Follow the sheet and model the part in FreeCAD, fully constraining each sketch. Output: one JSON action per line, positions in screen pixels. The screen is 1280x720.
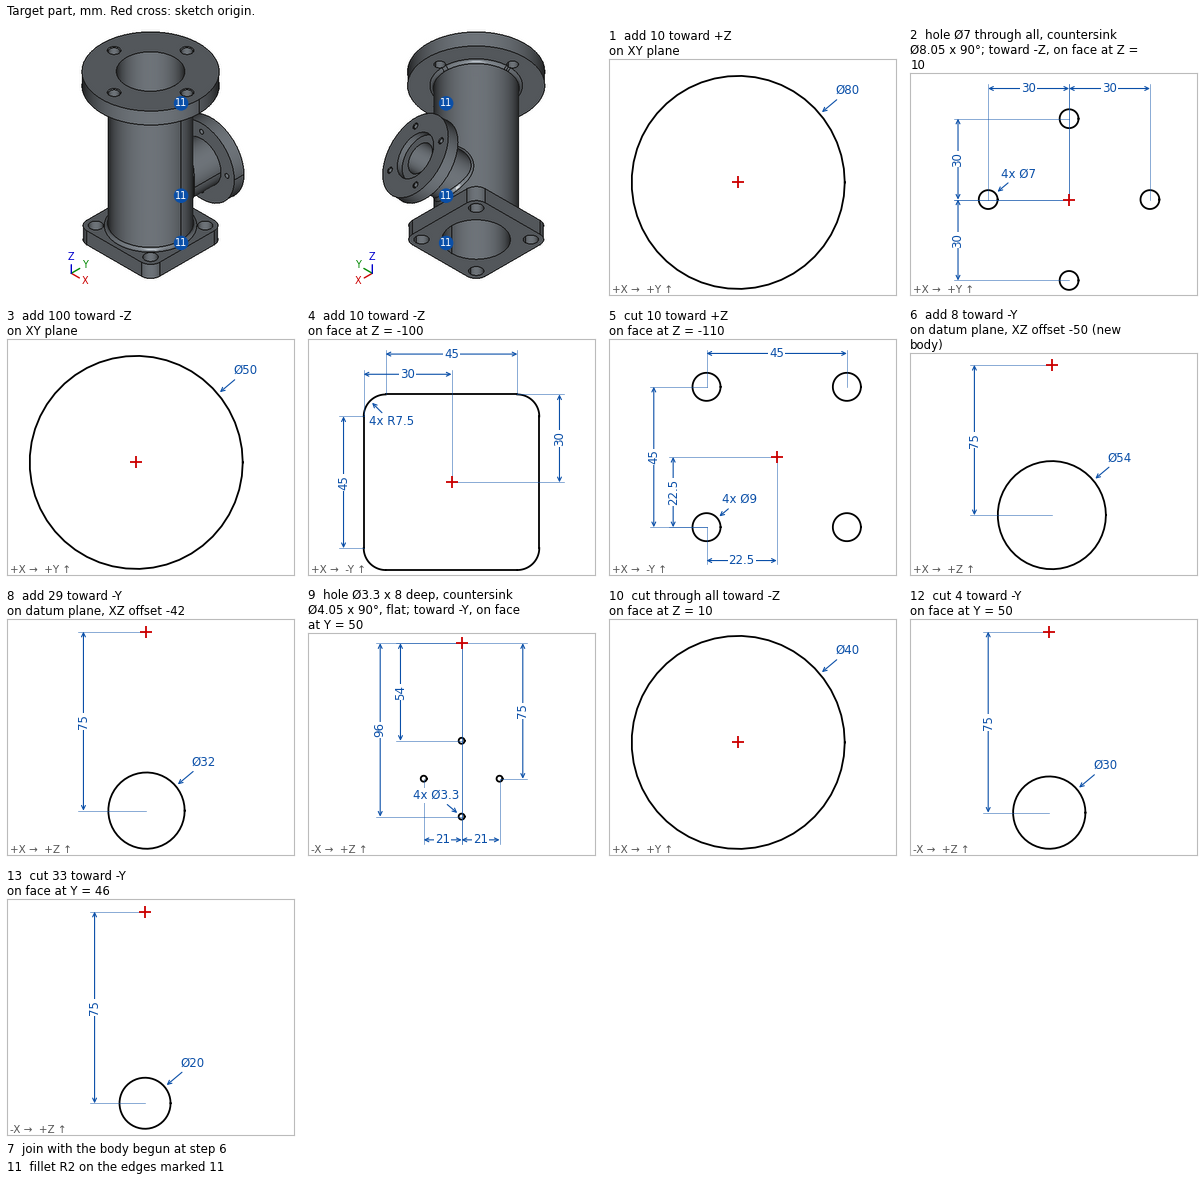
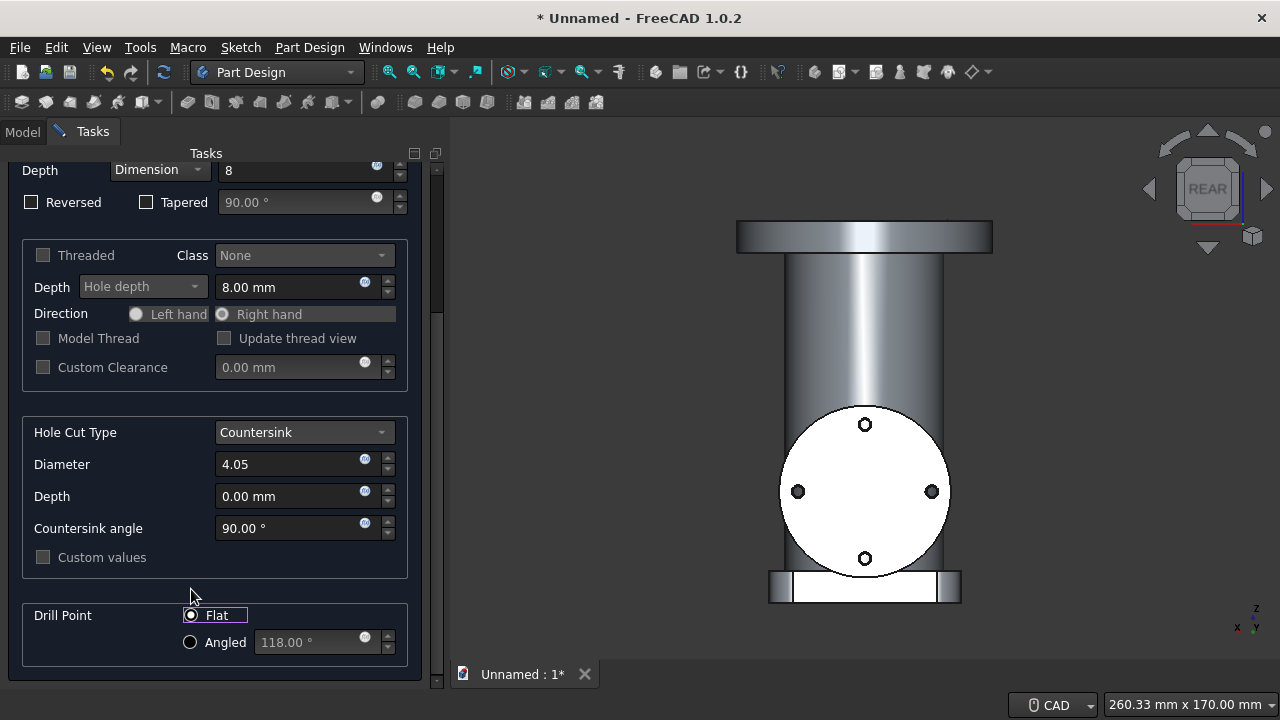
{"action": "scroll", "coordinate": [437, 426], "scroll_direction": "up", "scroll_amount": 5}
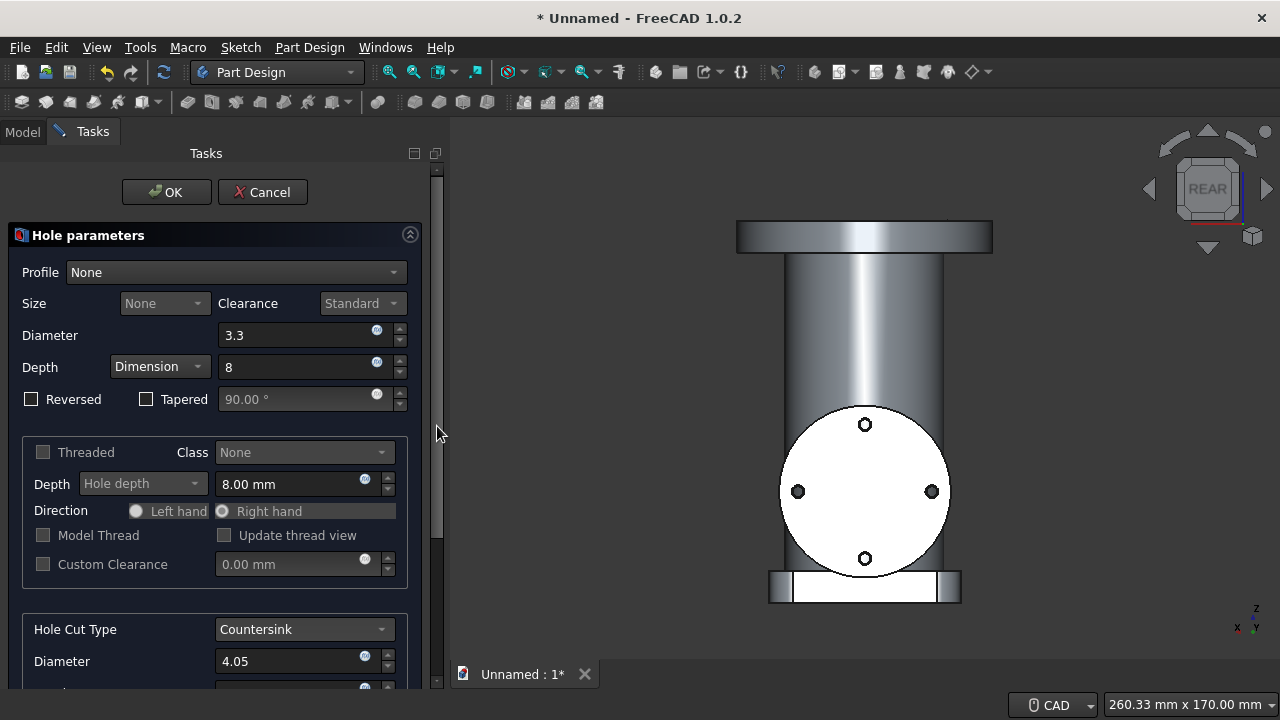
{"action": "left_click", "coordinate": [167, 192]}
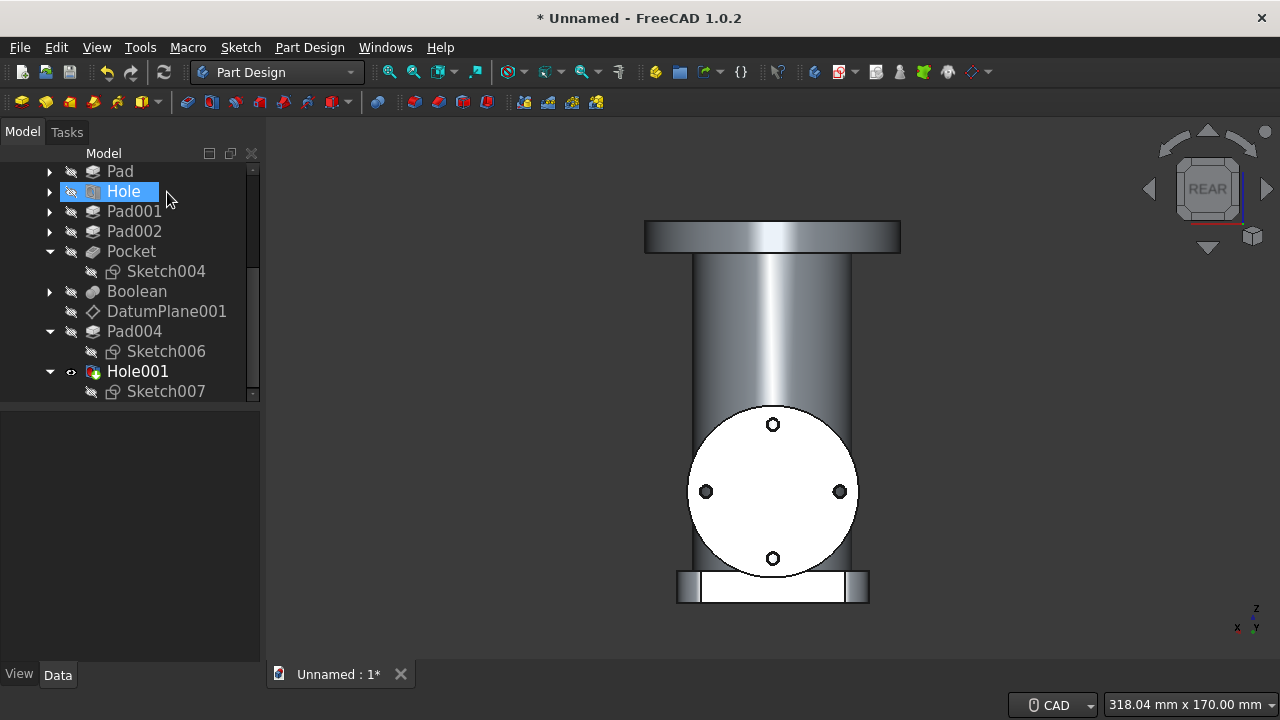
{"action": "key", "text": "0"}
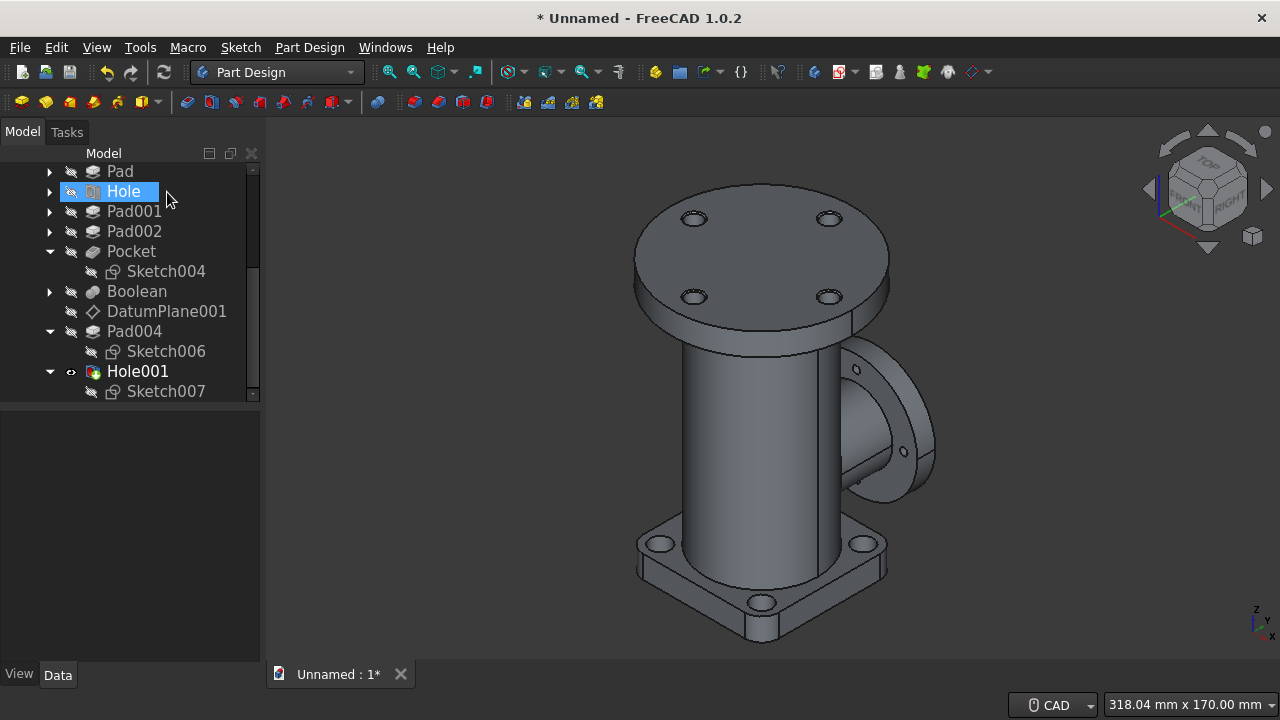
{"action": "left_click", "coordinate": [390, 72]}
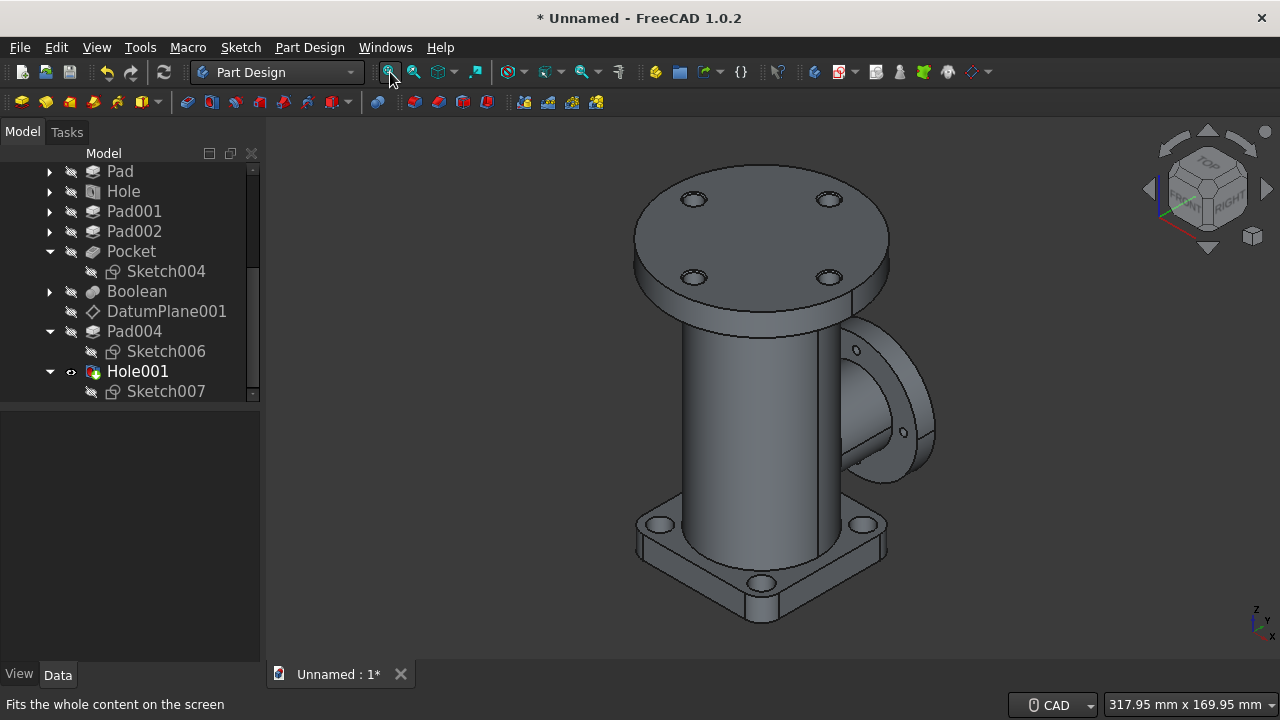
{"action": "left_click", "coordinate": [762, 237]}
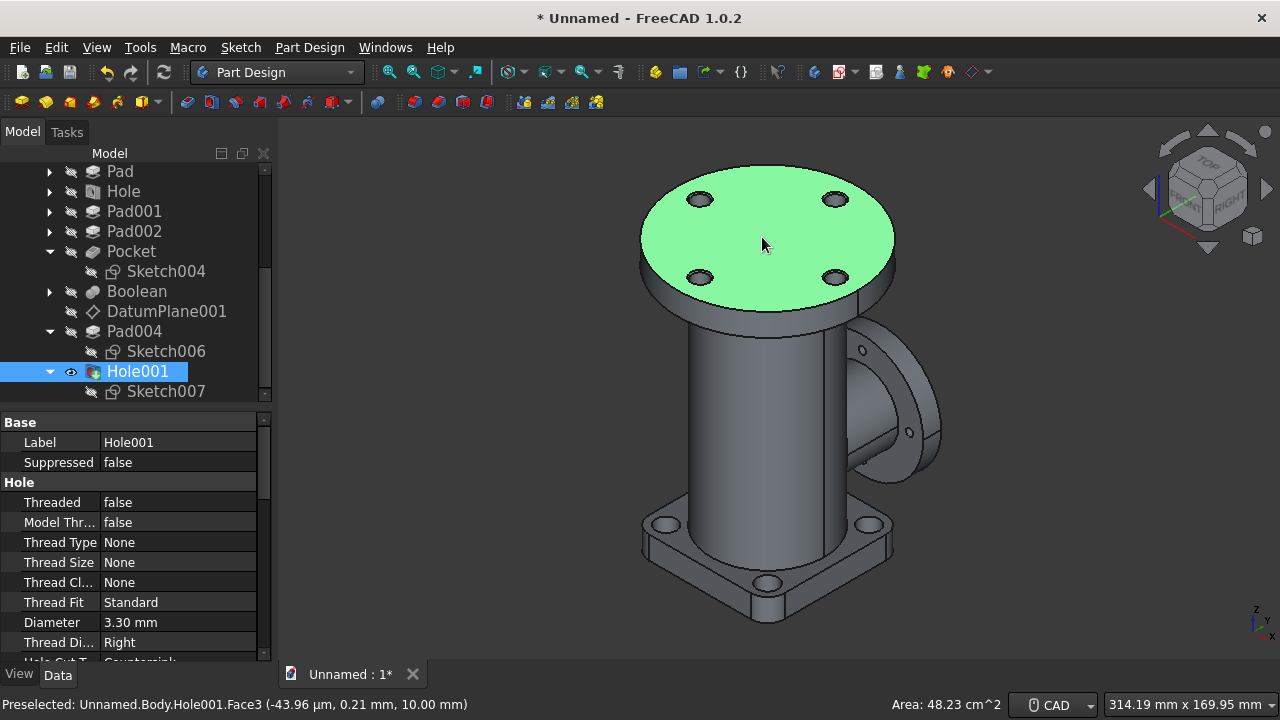
{"action": "left_click", "coordinate": [840, 72]}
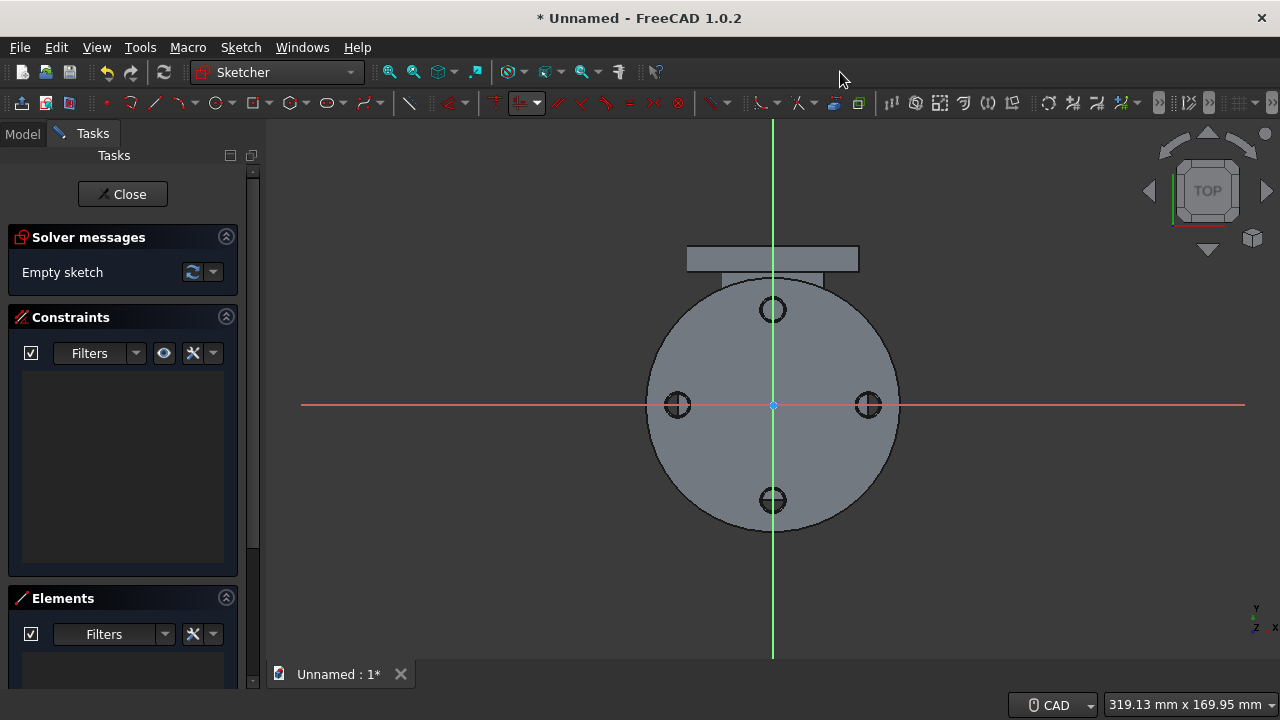
{"action": "scroll", "coordinate": [813, 414], "scroll_direction": "up", "scroll_amount": 5}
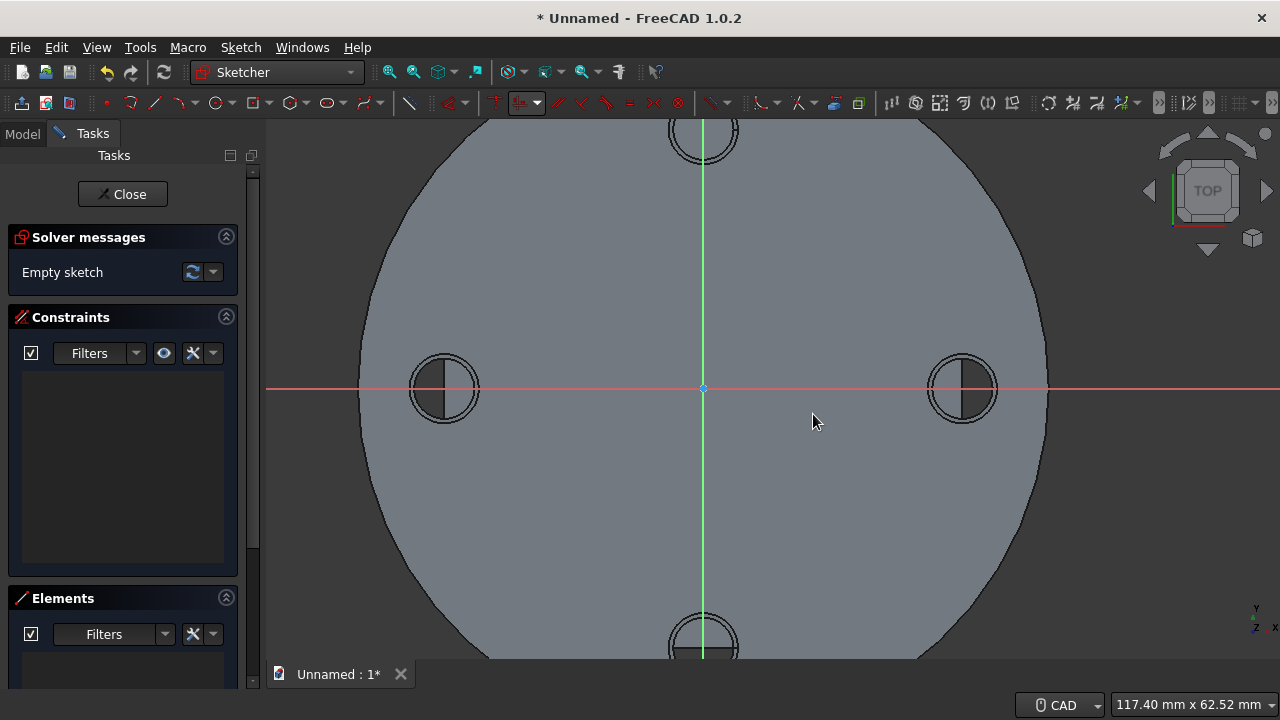
{"action": "left_click", "coordinate": [216, 104]}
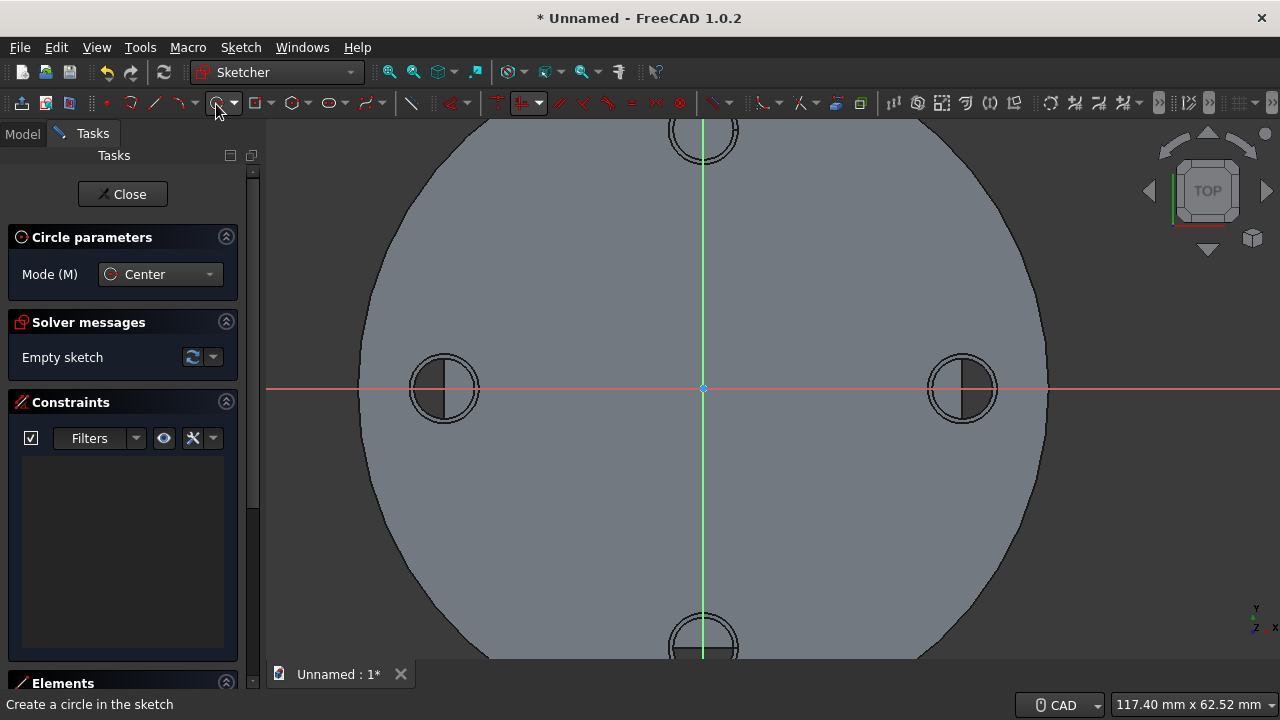
{"action": "left_click", "coordinate": [703, 389]}
{"action": "mouse_move", "coordinate": [825, 267]}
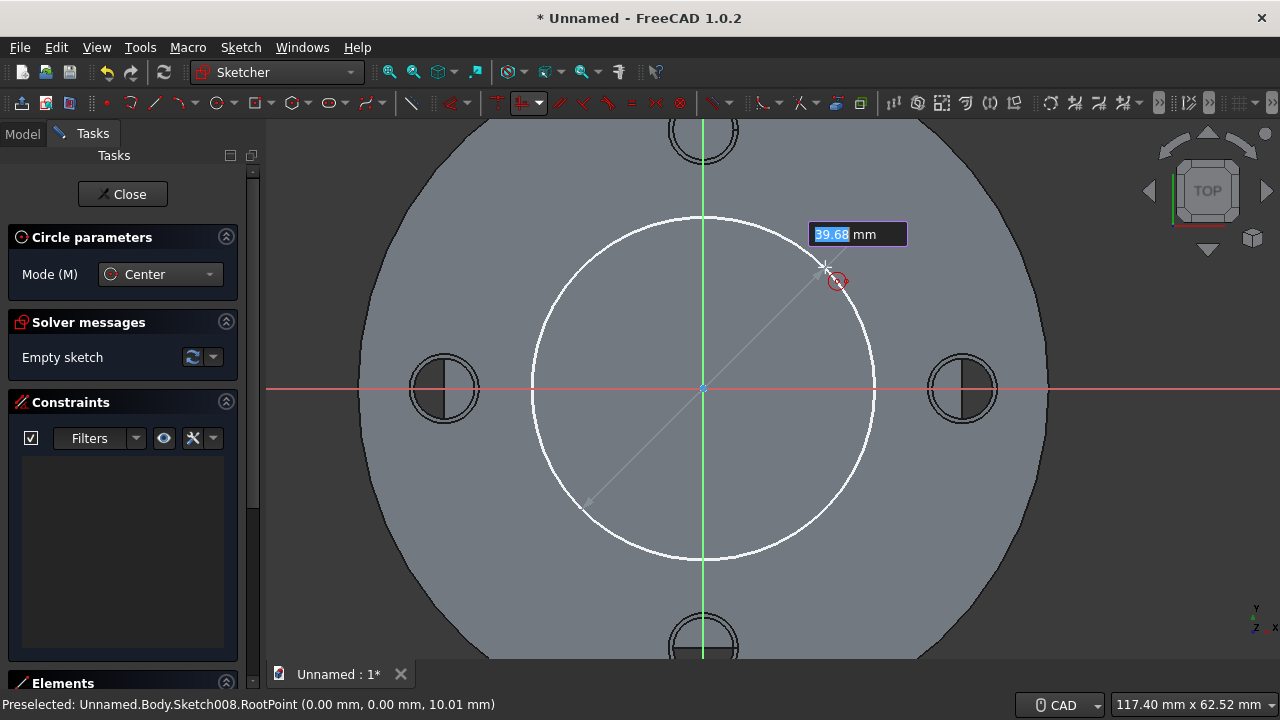
{"action": "type", "text": "40"}
{"action": "key", "text": "Return"}
{"action": "key", "text": "Escape"}